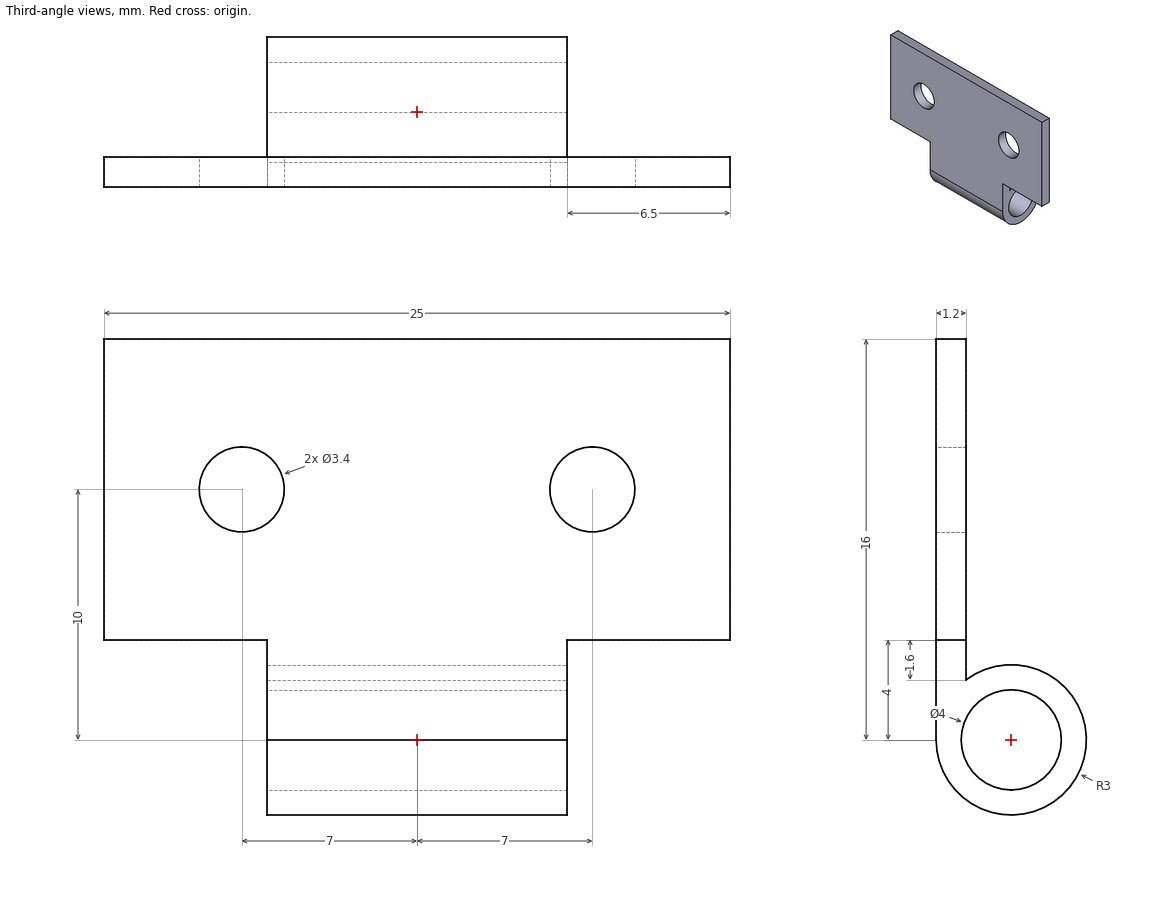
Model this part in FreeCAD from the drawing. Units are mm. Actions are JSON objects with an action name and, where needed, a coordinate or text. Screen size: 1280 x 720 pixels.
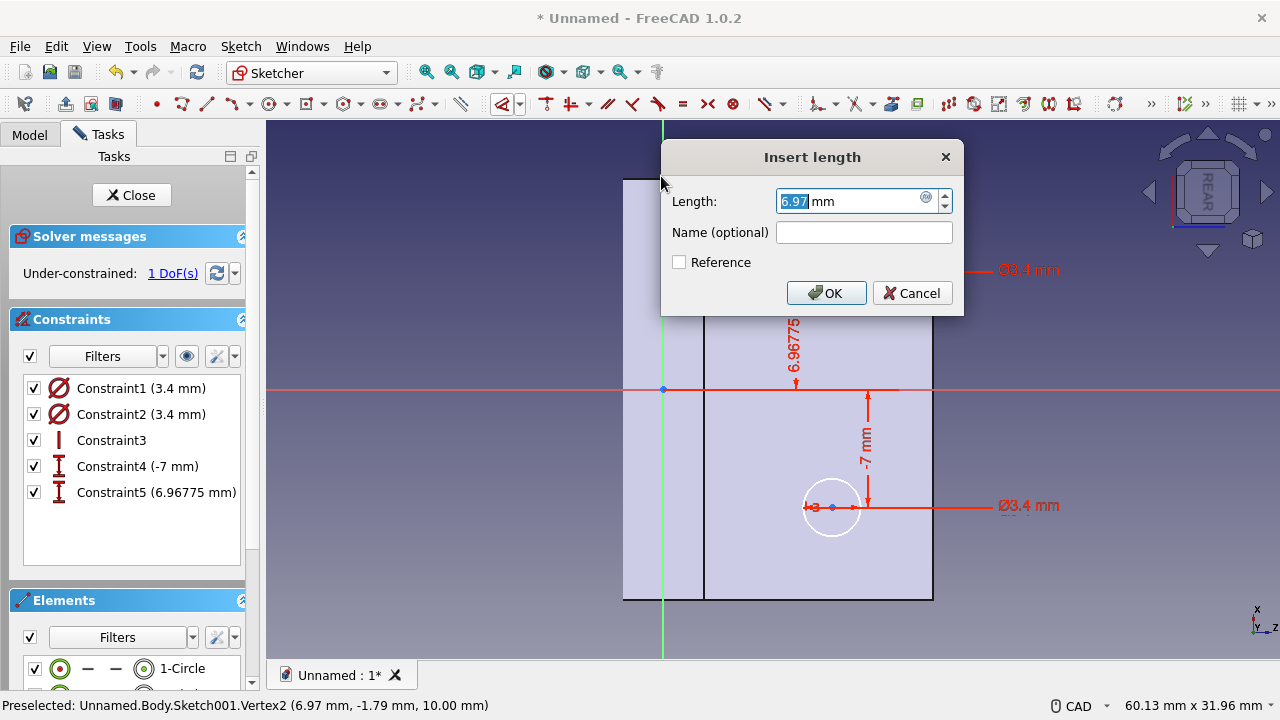
{"action": "type", "text": "7"}
{"action": "key", "text": "Return"}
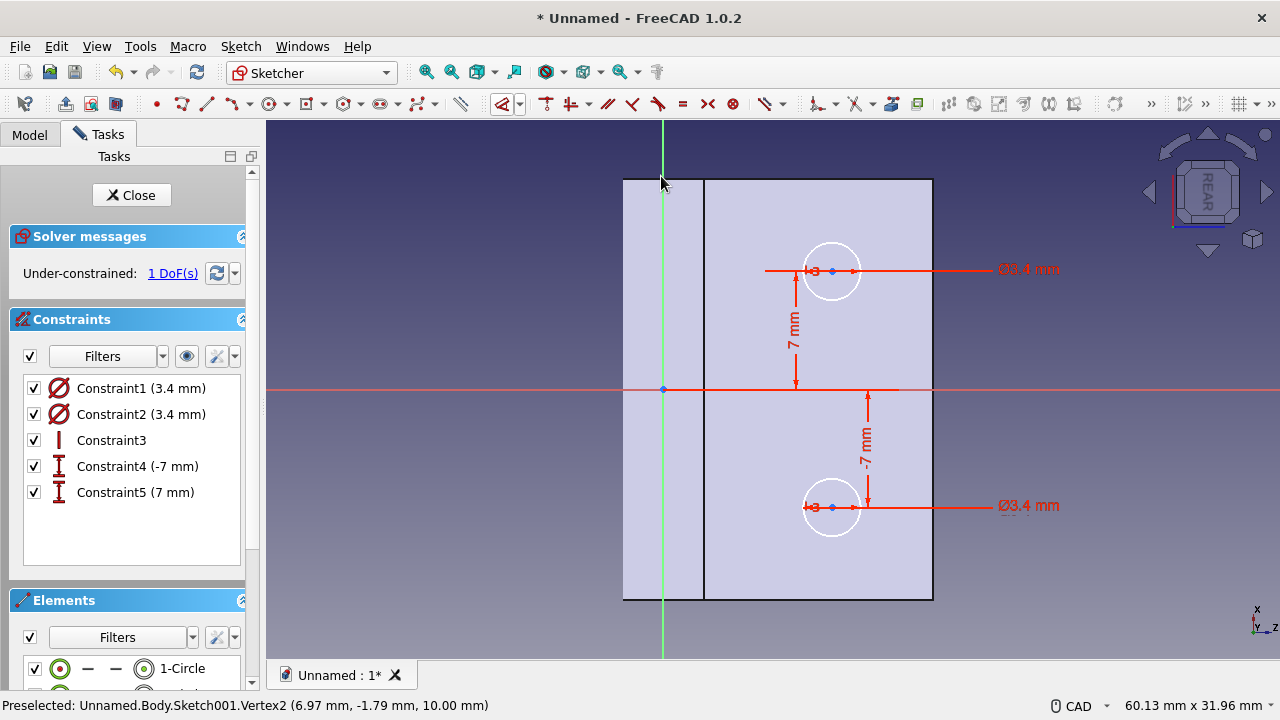
{"action": "left_click", "coordinate": [832, 508]}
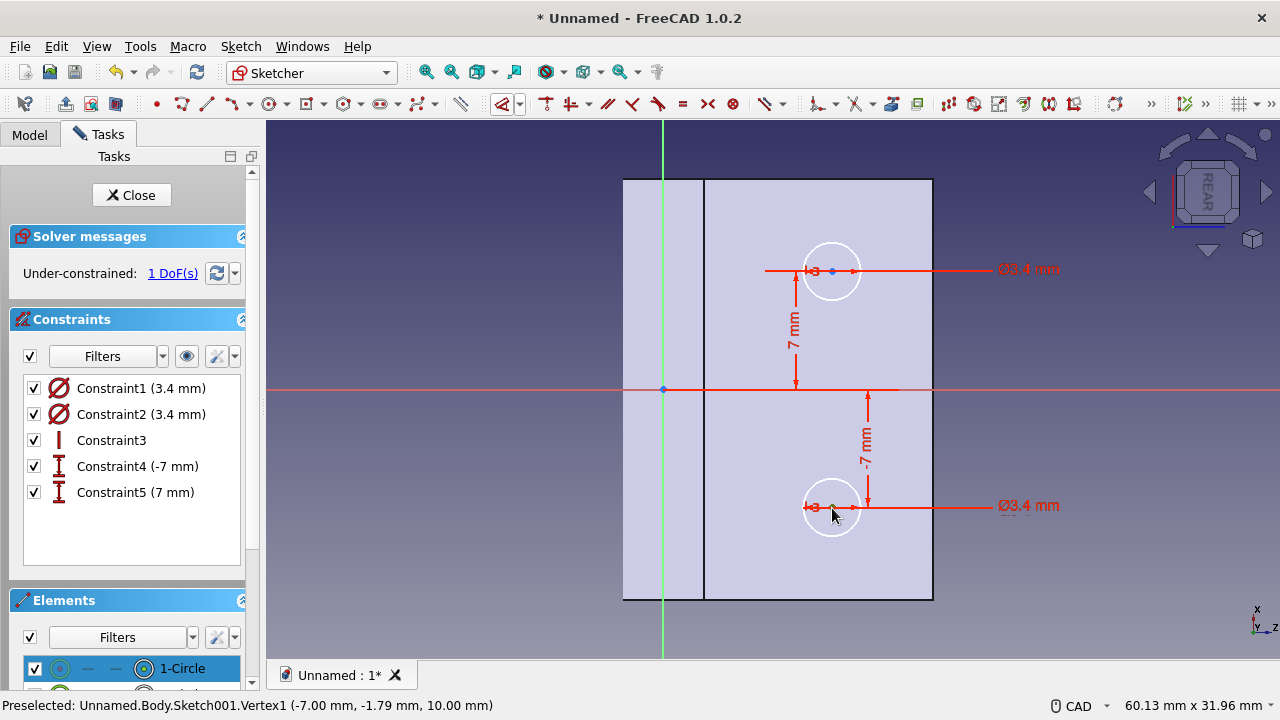
{"action": "key", "text": "l"}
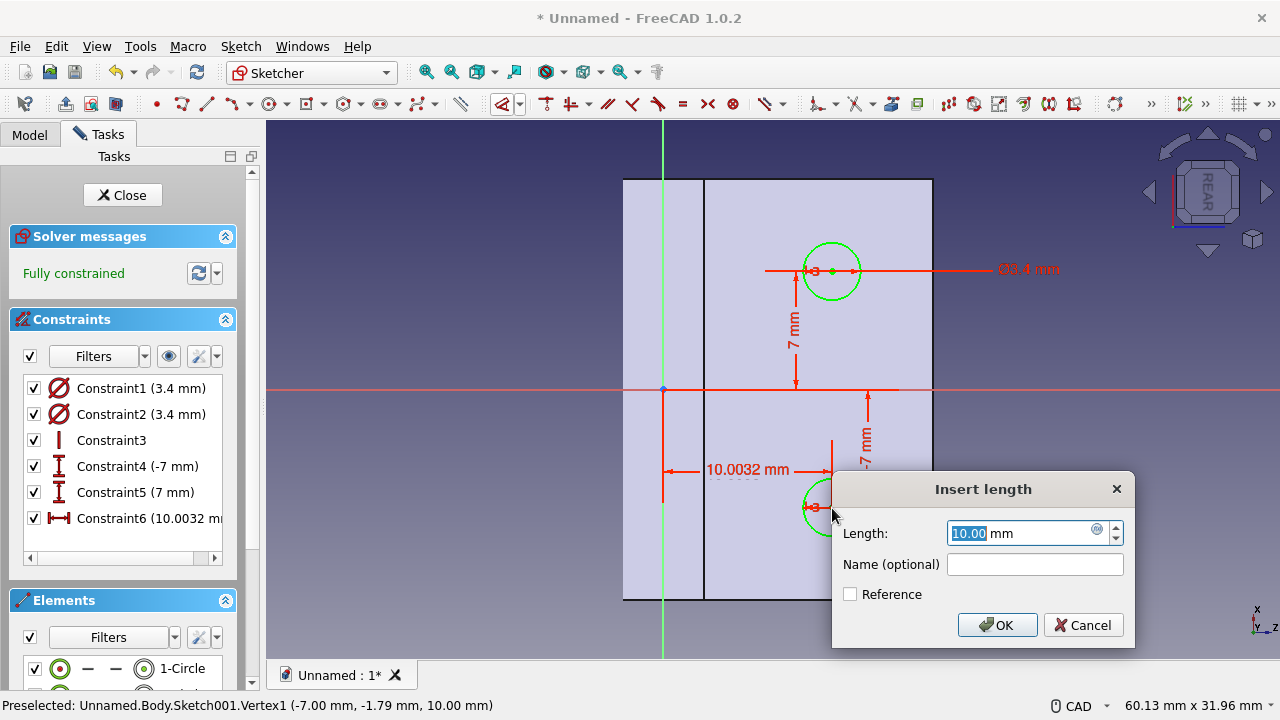
{"action": "type", "text": "10"}
{"action": "key", "text": "Return"}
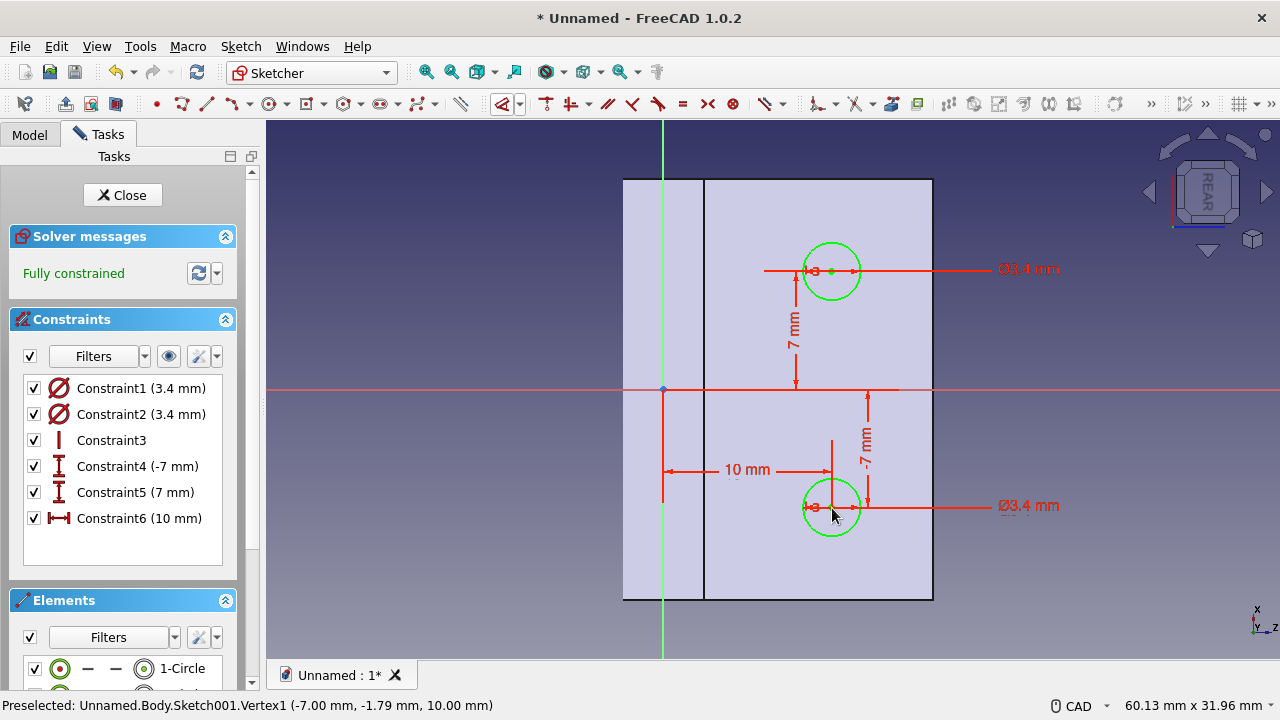
{"action": "left_click", "coordinate": [123, 195]}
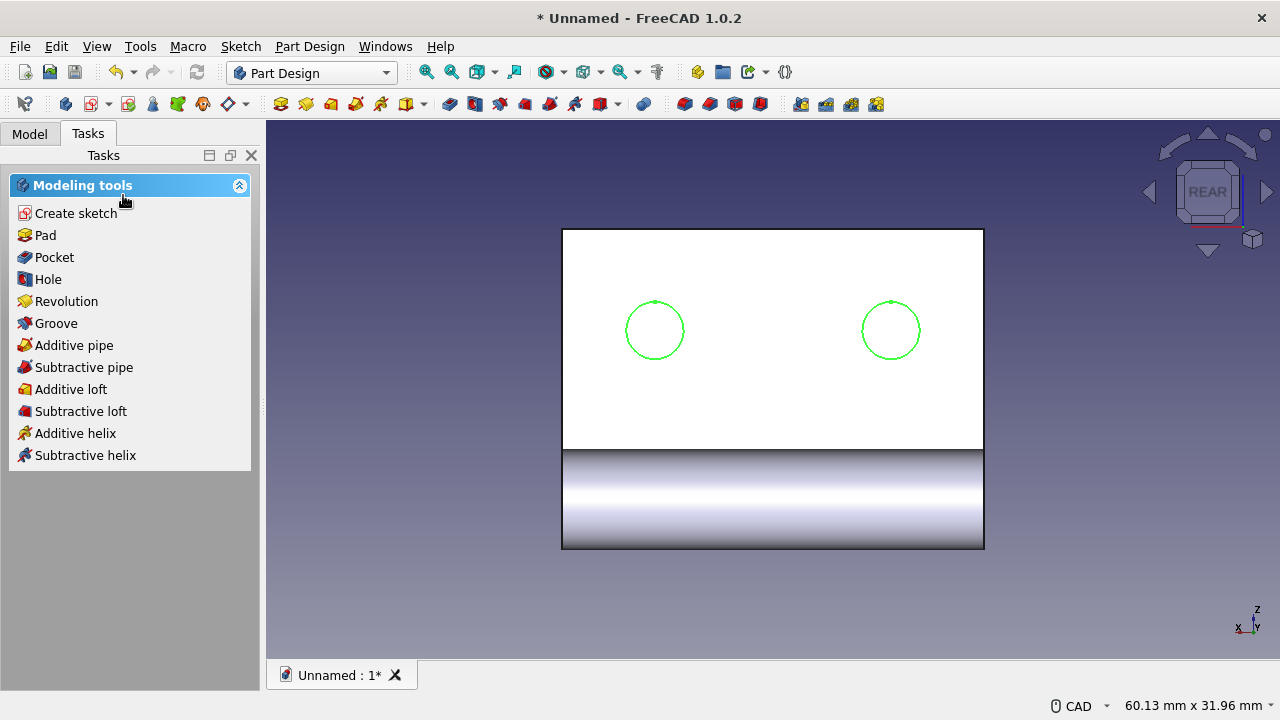
{"action": "left_click", "coordinate": [450, 104]}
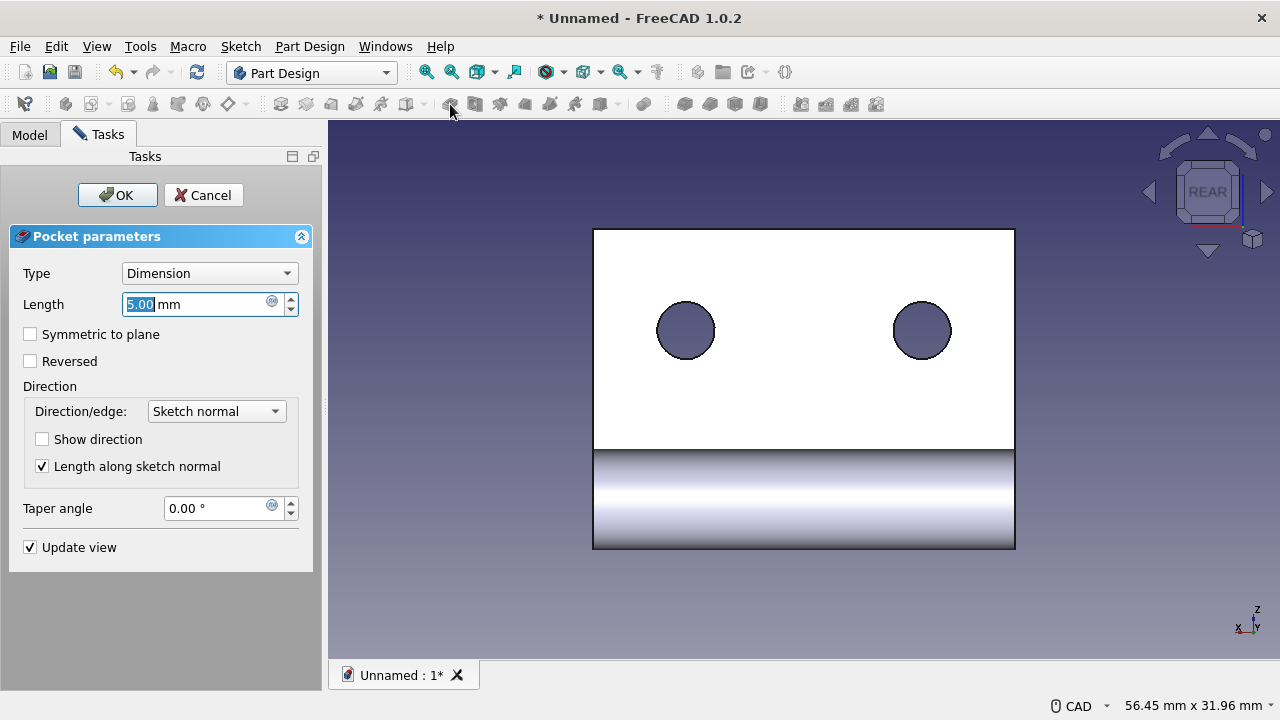
{"action": "left_click", "coordinate": [210, 274]}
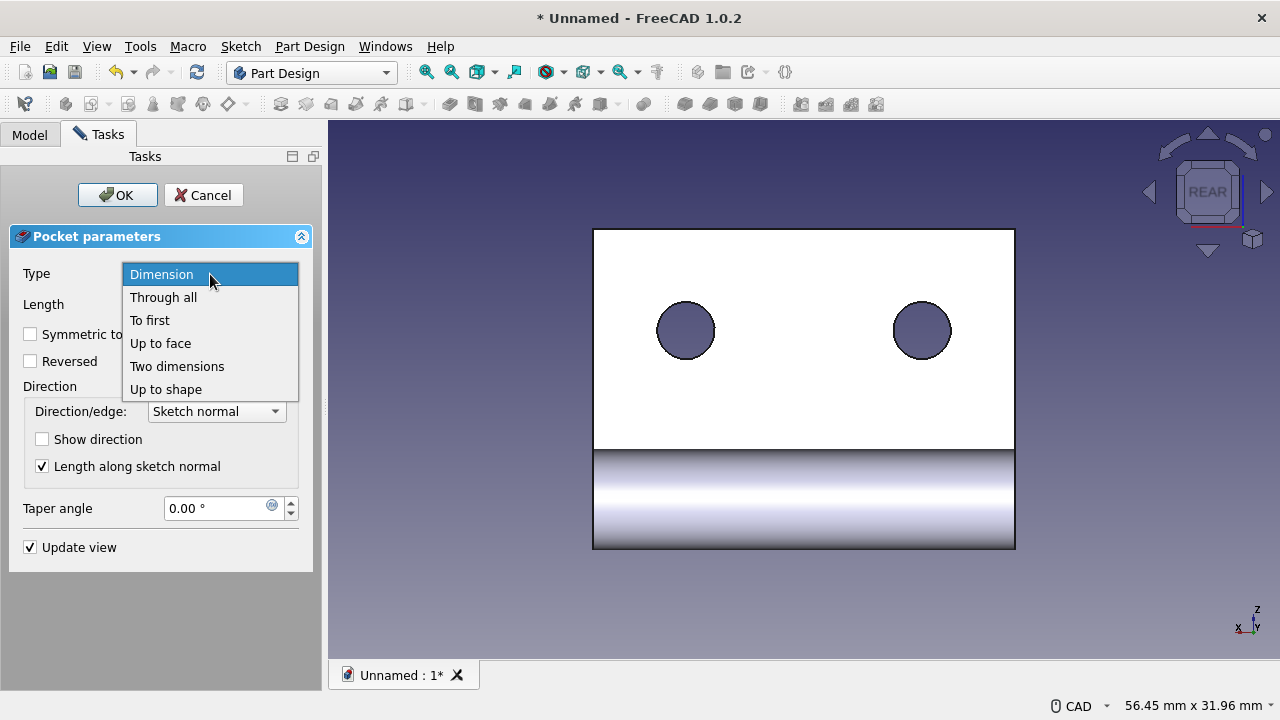
{"action": "left_click", "coordinate": [208, 298]}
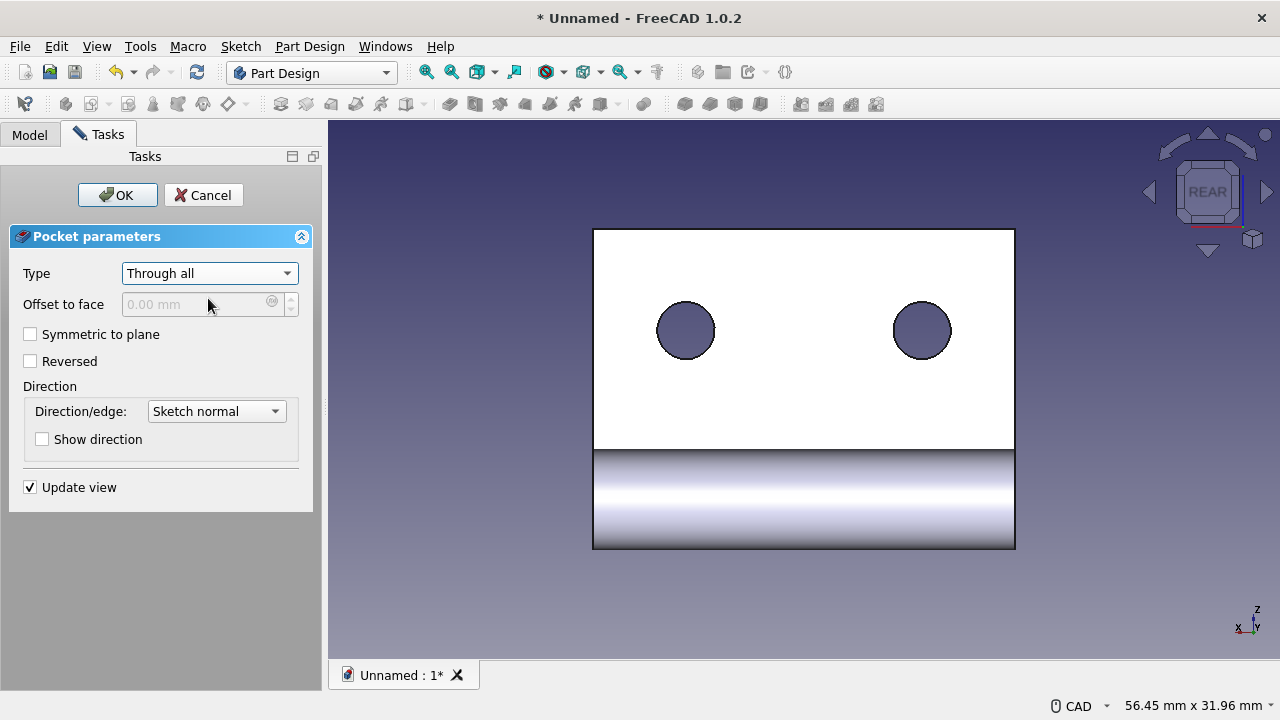
{"action": "left_click", "coordinate": [118, 195]}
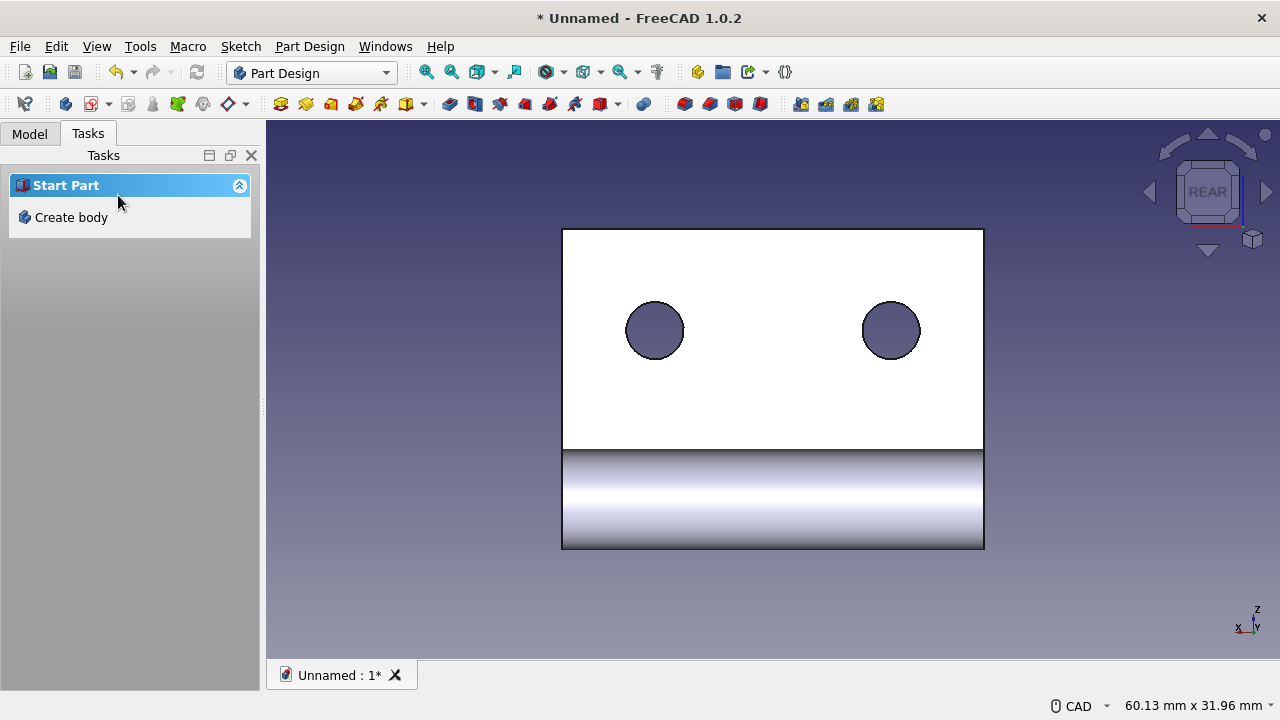
{"action": "key", "text": "0"}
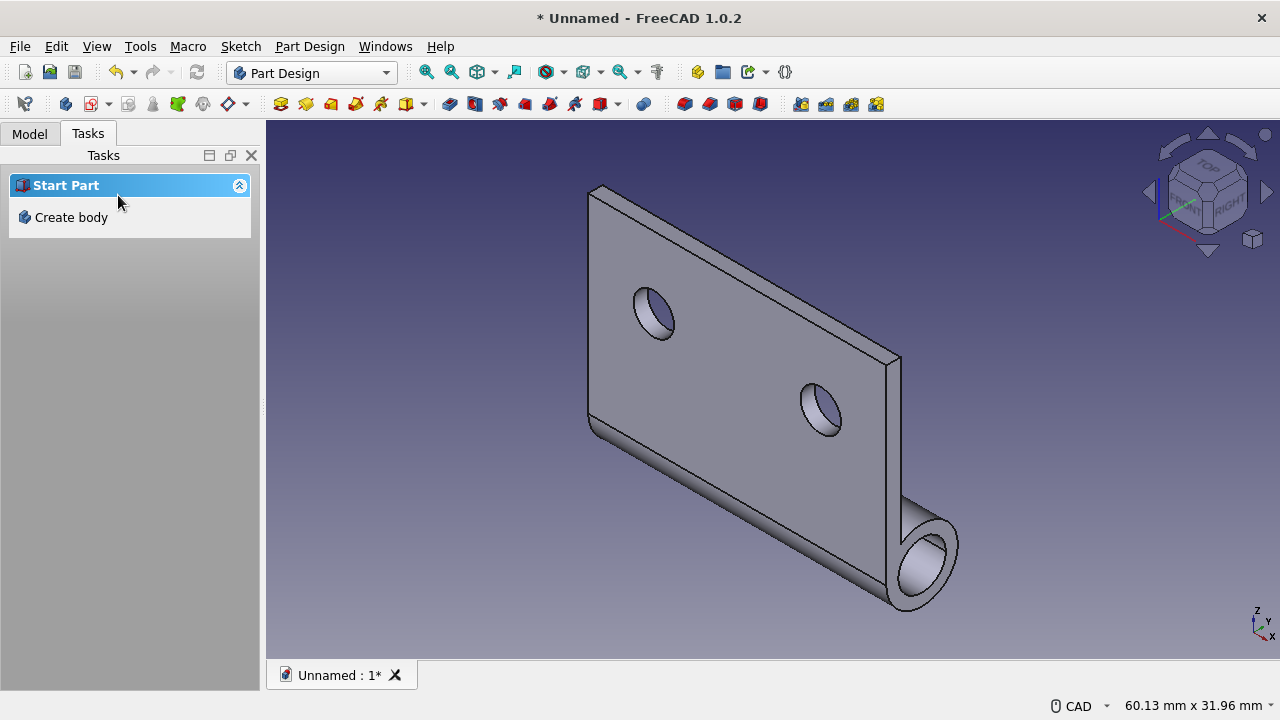
{"action": "key", "text": "3"}